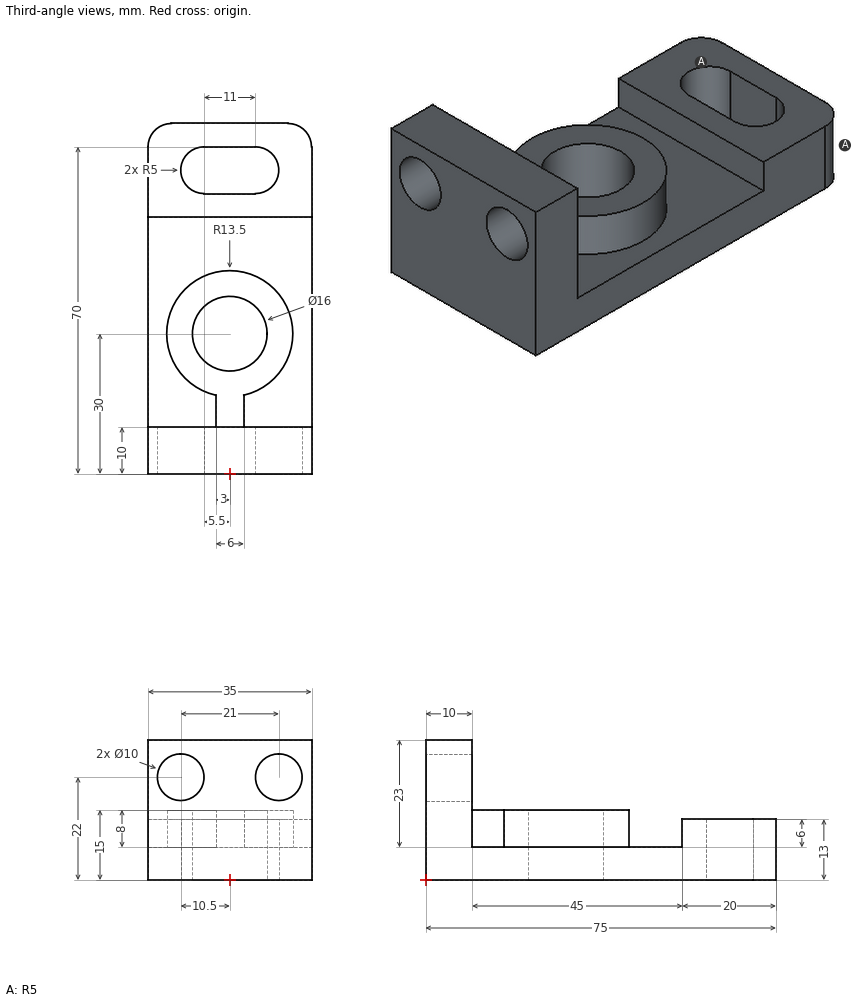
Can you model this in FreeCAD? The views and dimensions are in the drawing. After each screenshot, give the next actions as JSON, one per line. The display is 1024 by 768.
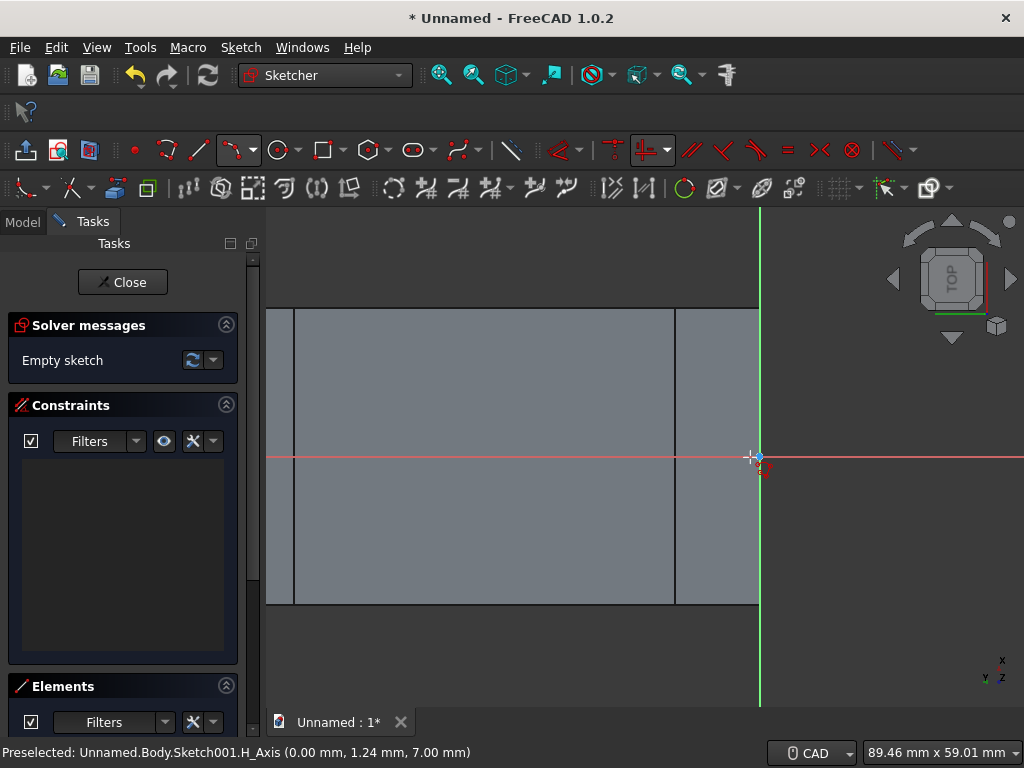
{"action": "left_click", "coordinate": [617, 482]}
{"action": "left_click", "coordinate": [675, 482]}
{"action": "left_click", "coordinate": [675, 431]}
{"action": "left_click", "coordinate": [617, 431]}
{"action": "right_click", "coordinate": [617, 431]}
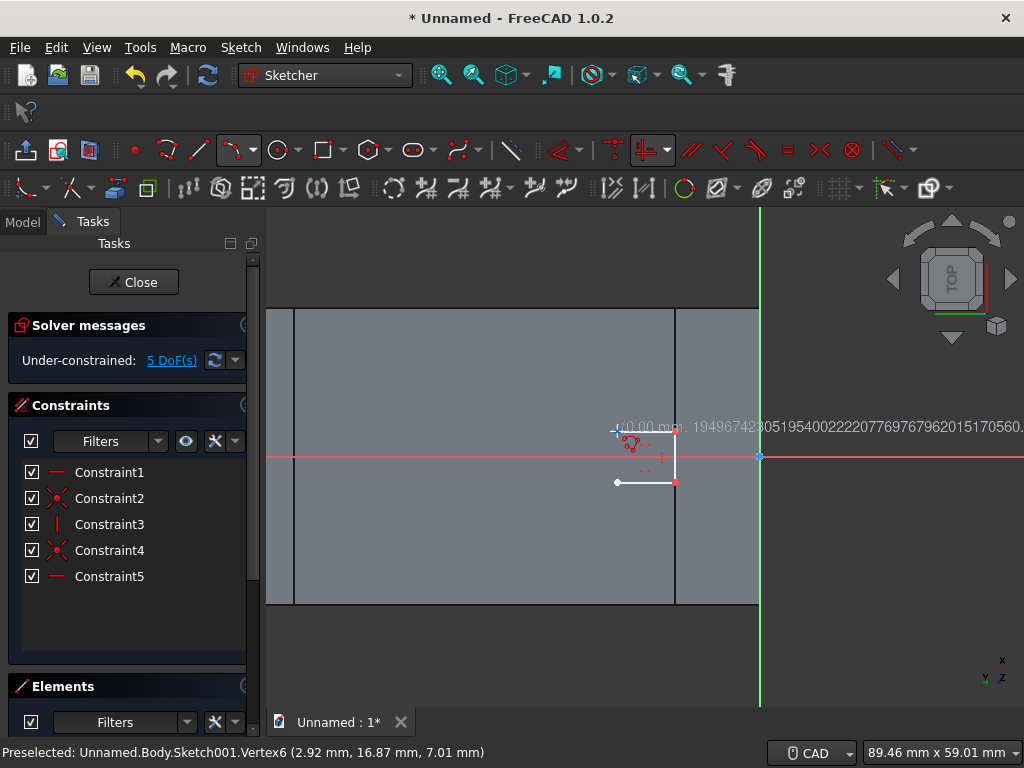
{"action": "left_click", "coordinate": [232, 150]}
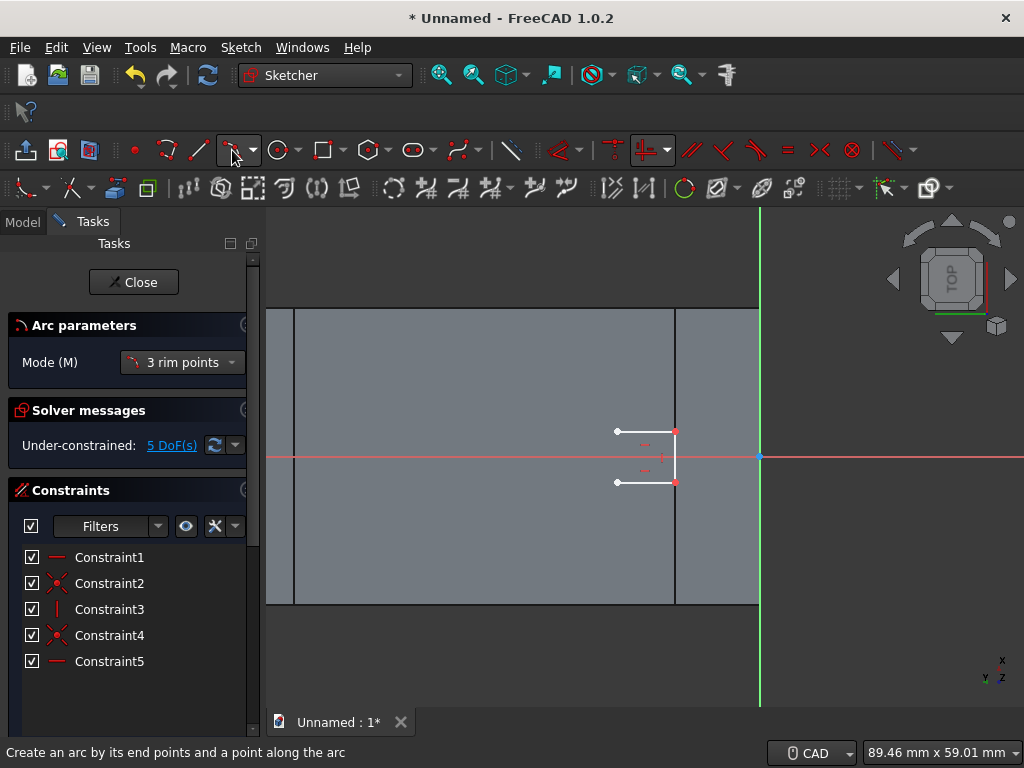
{"action": "left_click", "coordinate": [617, 432]}
{"action": "left_click", "coordinate": [617, 483]}
{"action": "left_click", "coordinate": [410, 394]}
{"action": "key", "text": "Escape"}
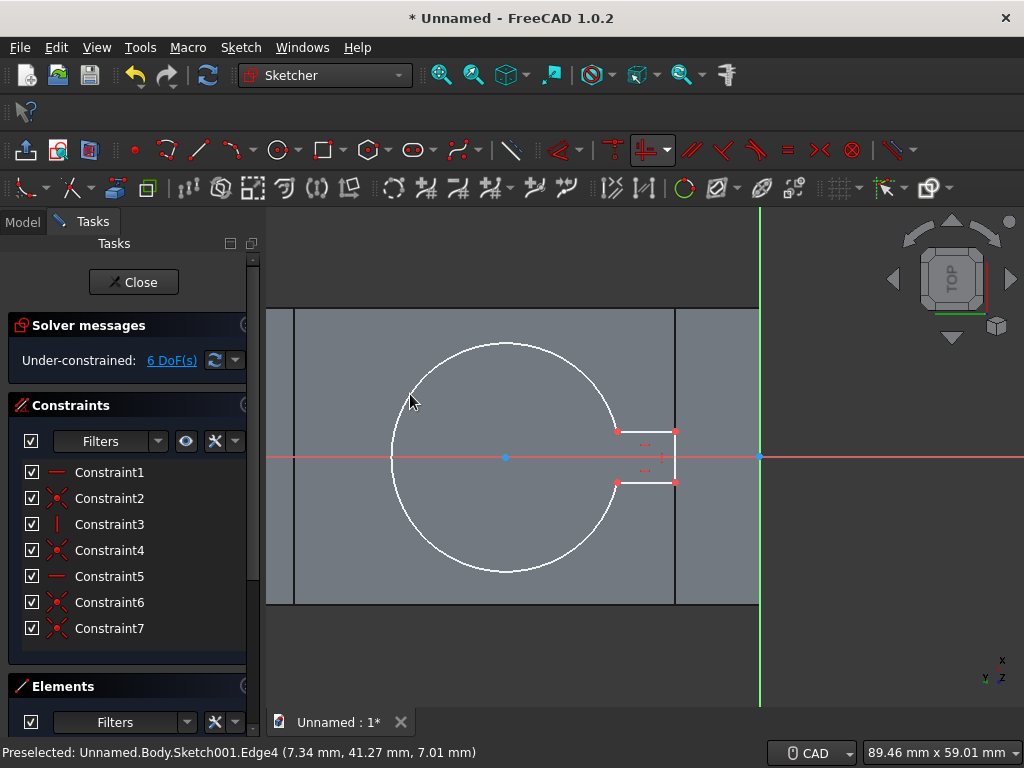
{"action": "left_click", "coordinate": [506, 457]}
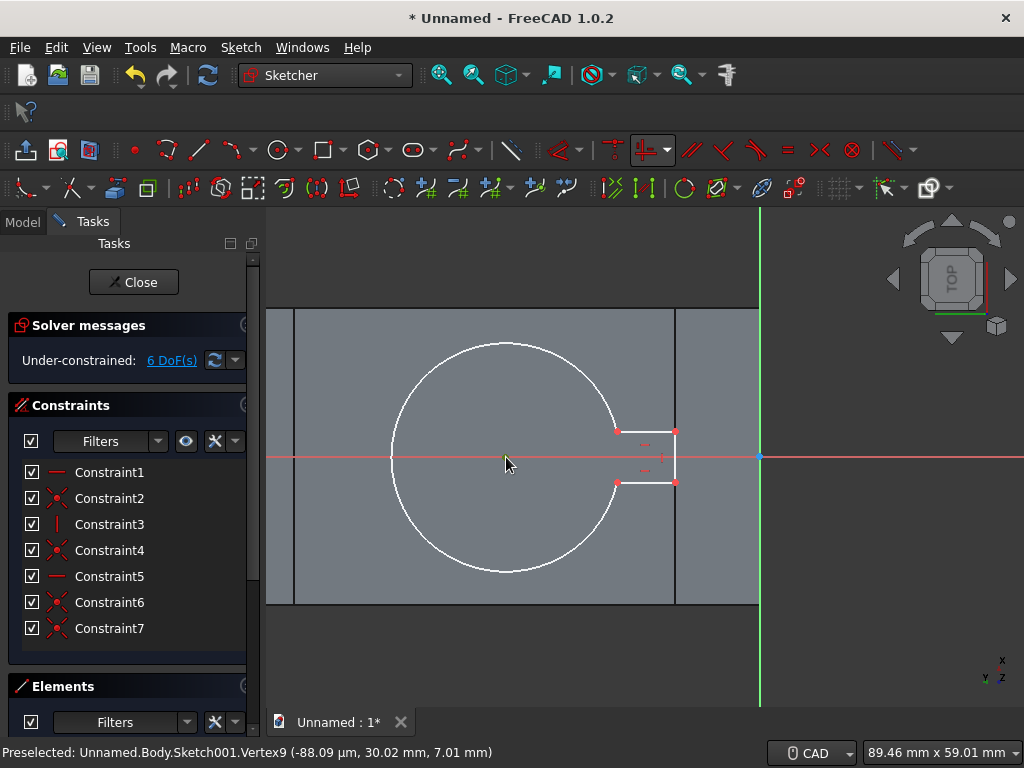
{"action": "left_click", "coordinate": [334, 457]}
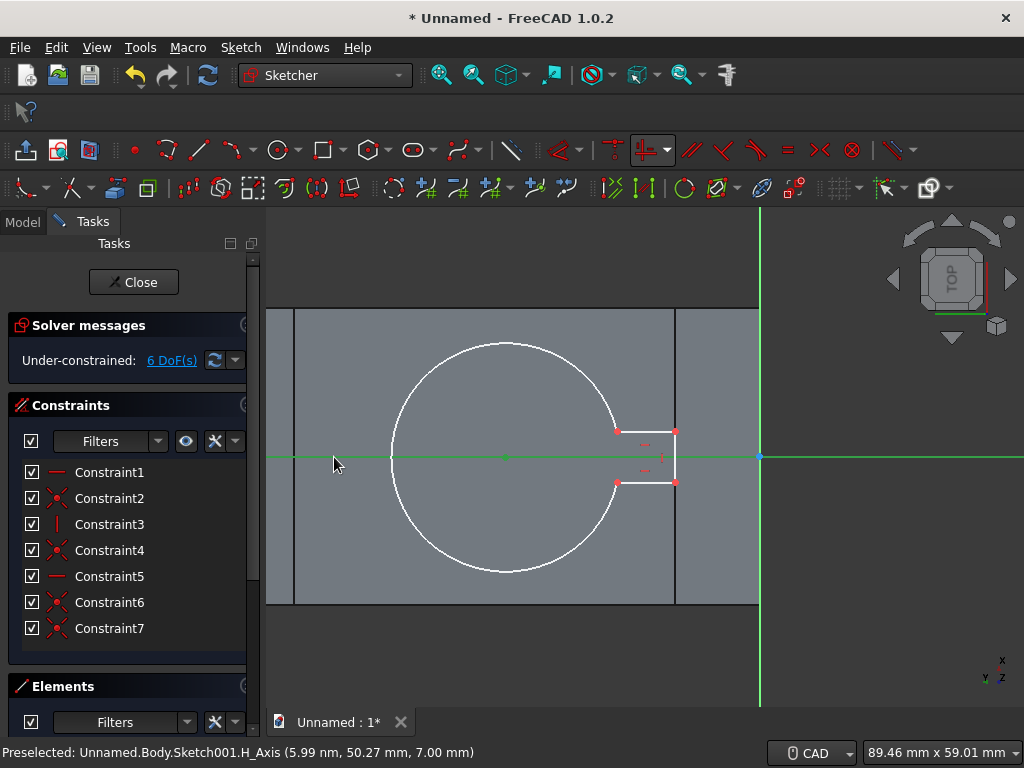
{"action": "key", "text": "c"}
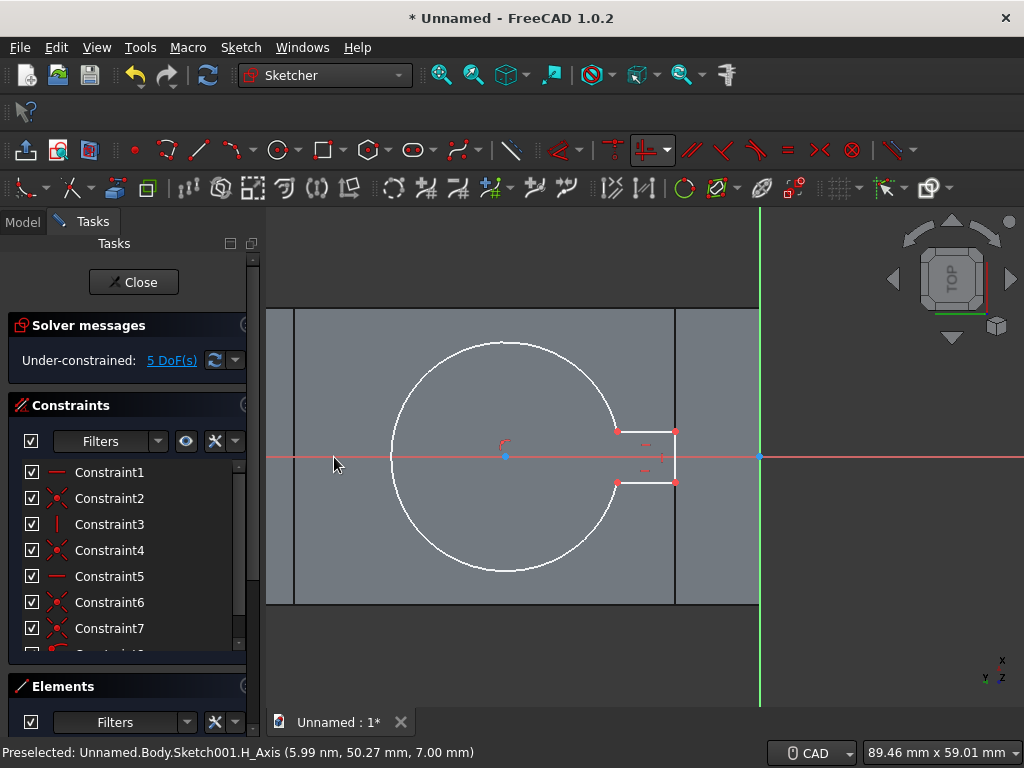
{"action": "left_click", "coordinate": [558, 150]}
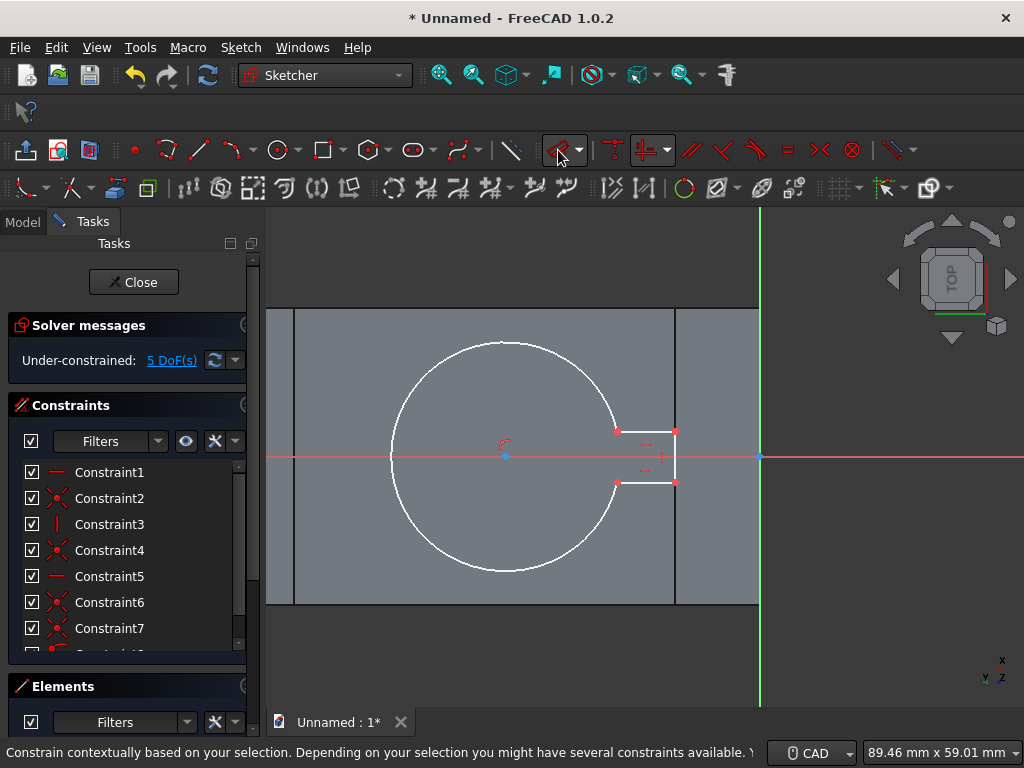
{"action": "left_click", "coordinate": [461, 351]}
{"action": "left_click", "coordinate": [449, 322]}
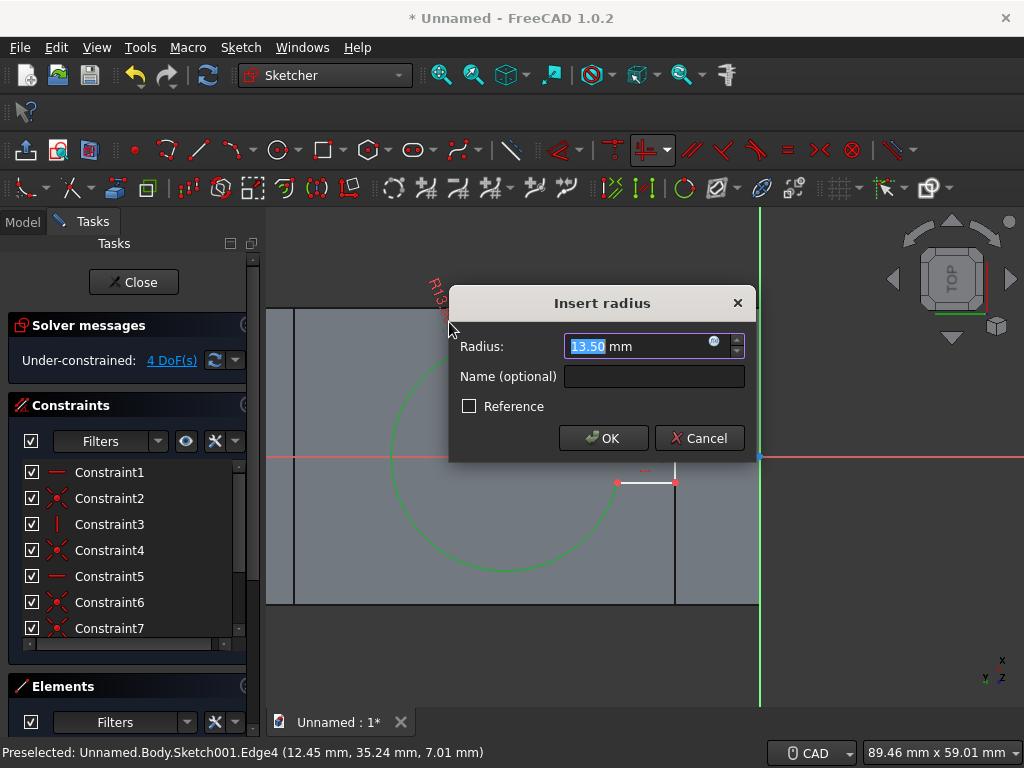
{"action": "type", "text": "13.5"}
{"action": "key", "text": "Return"}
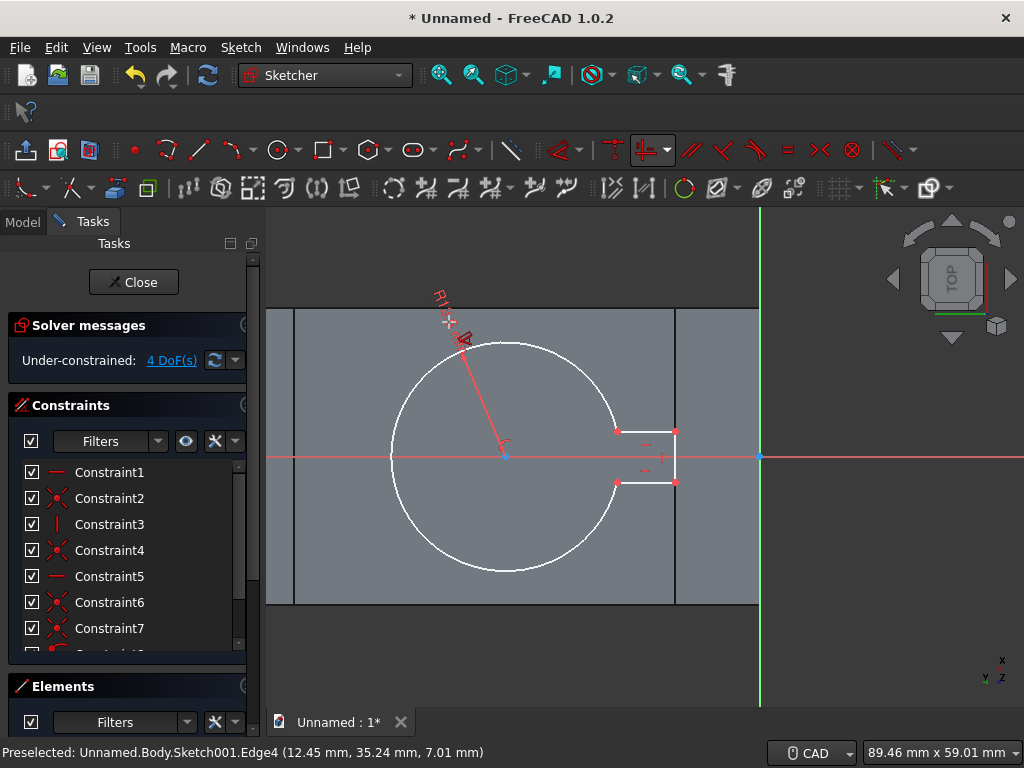
{"action": "scroll", "coordinate": [675, 468], "scroll_direction": "up", "scroll_amount": 2}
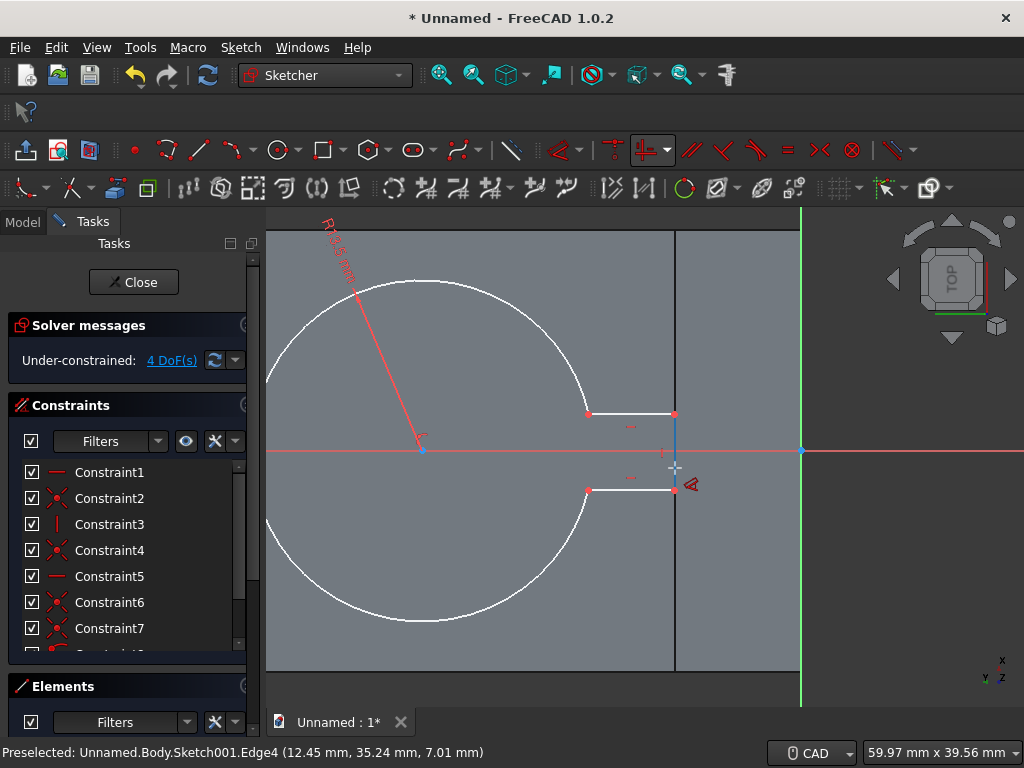
{"action": "left_click", "coordinate": [675, 467]}
{"action": "left_click", "coordinate": [709, 435]}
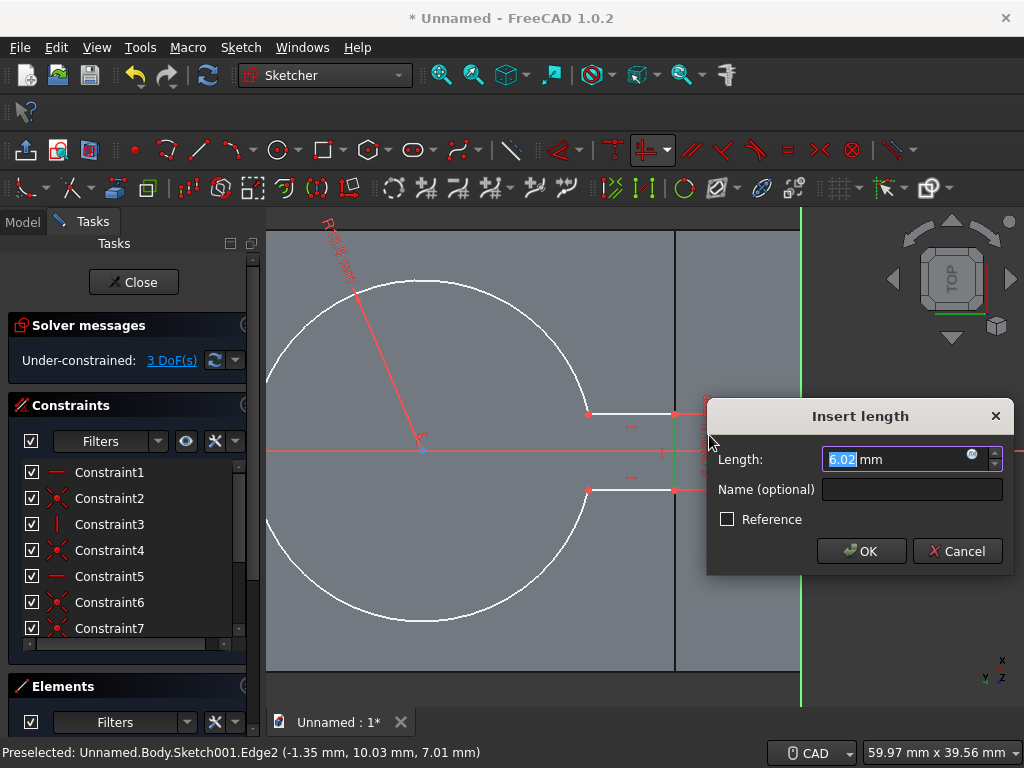
{"action": "type", "text": "6"}
{"action": "key", "text": "Return"}